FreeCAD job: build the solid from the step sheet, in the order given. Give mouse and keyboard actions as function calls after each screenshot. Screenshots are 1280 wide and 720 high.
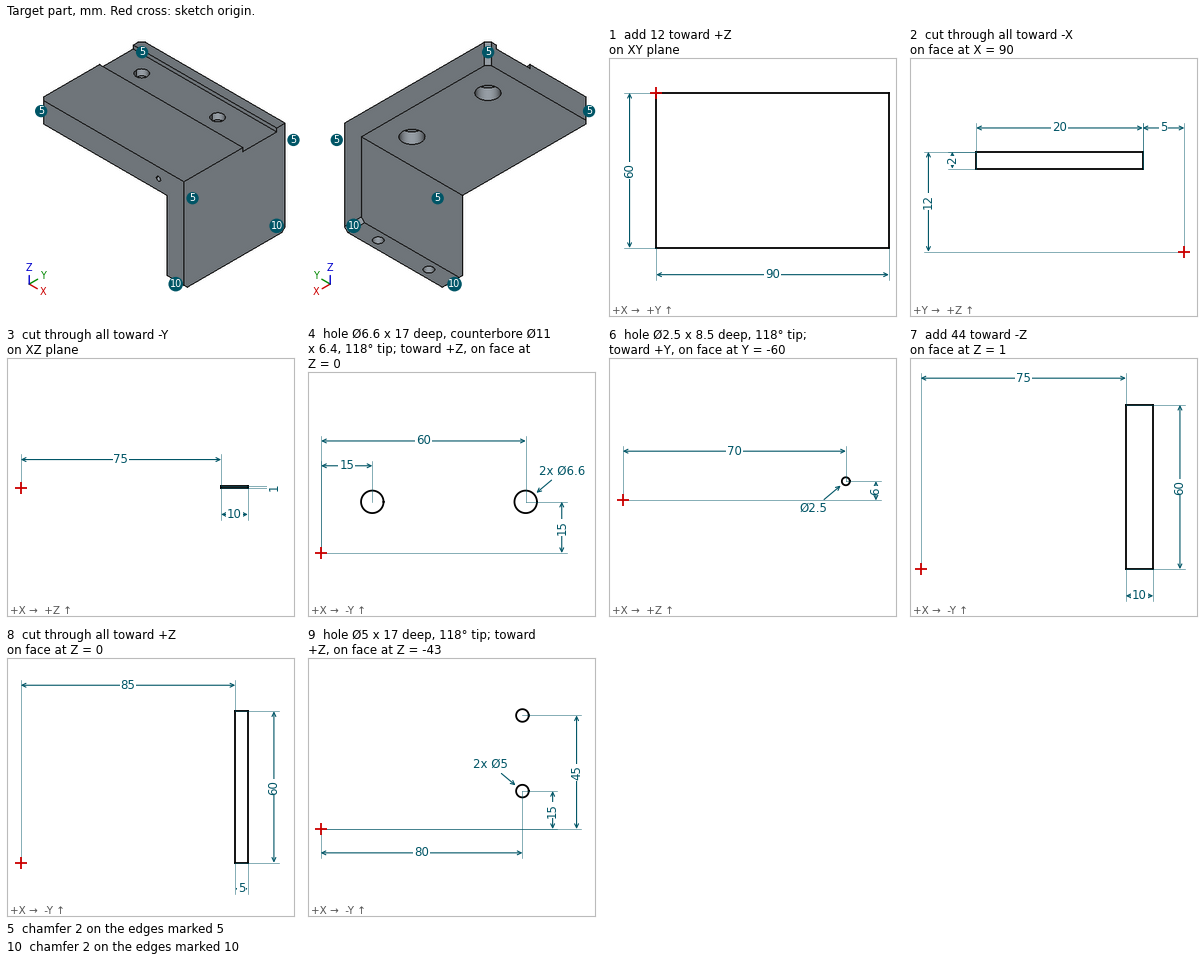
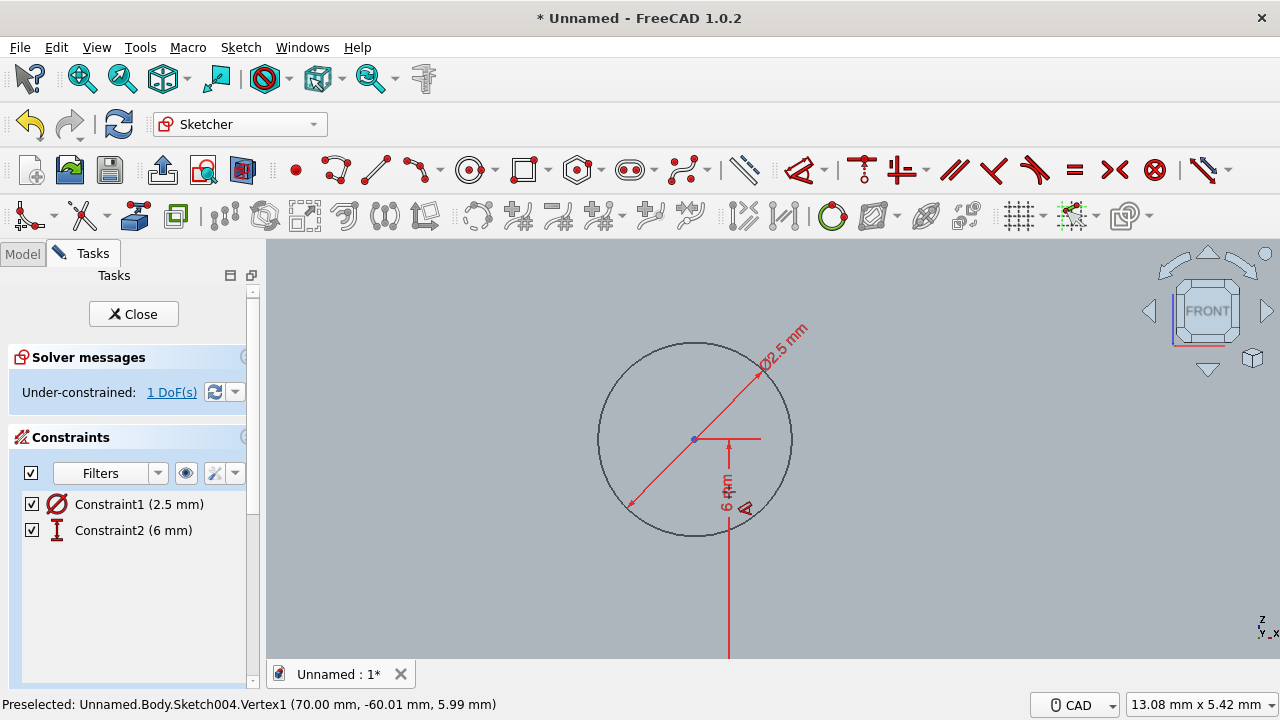
click(695, 439)
click(494, 405)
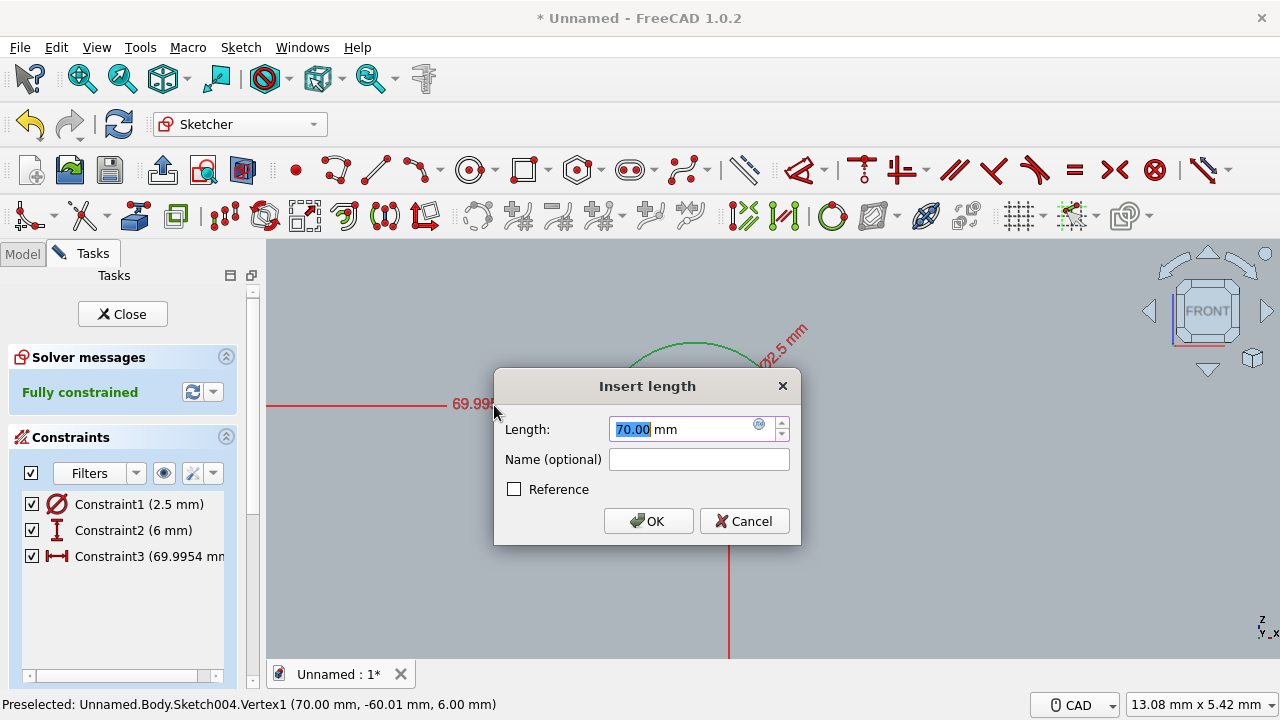
text(70)
key(Return)
key(Escape)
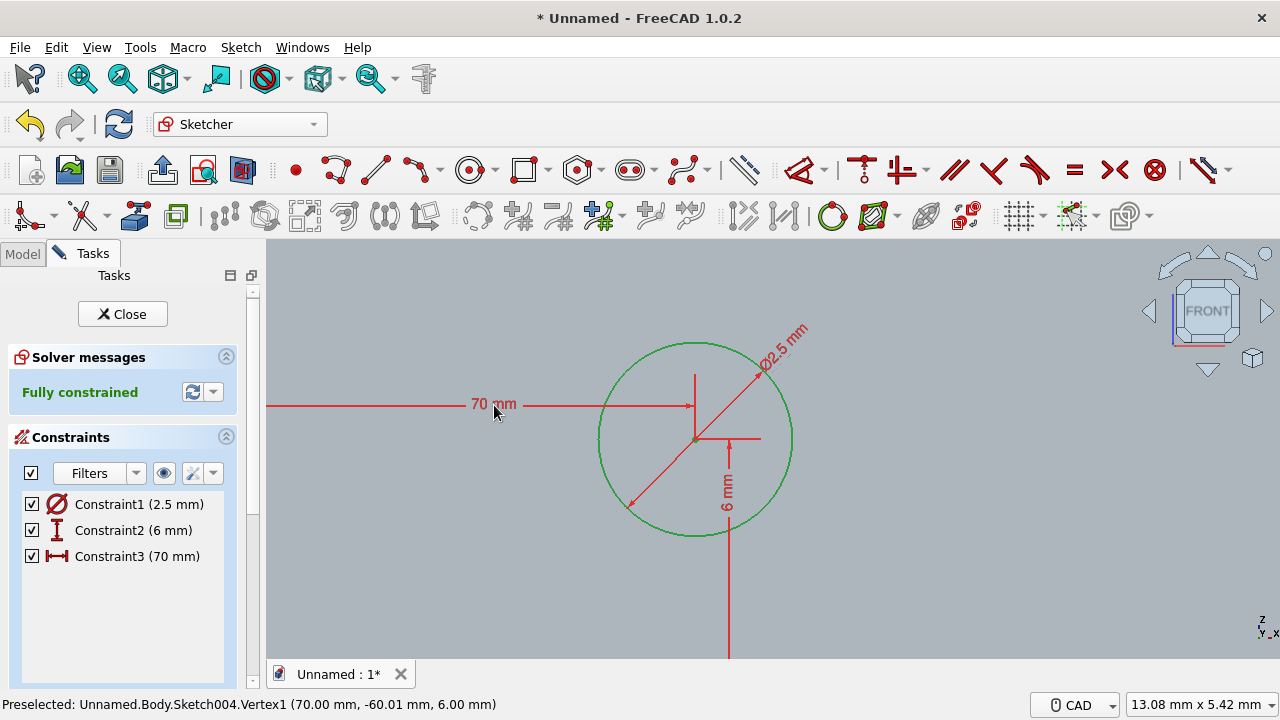
click(123, 314)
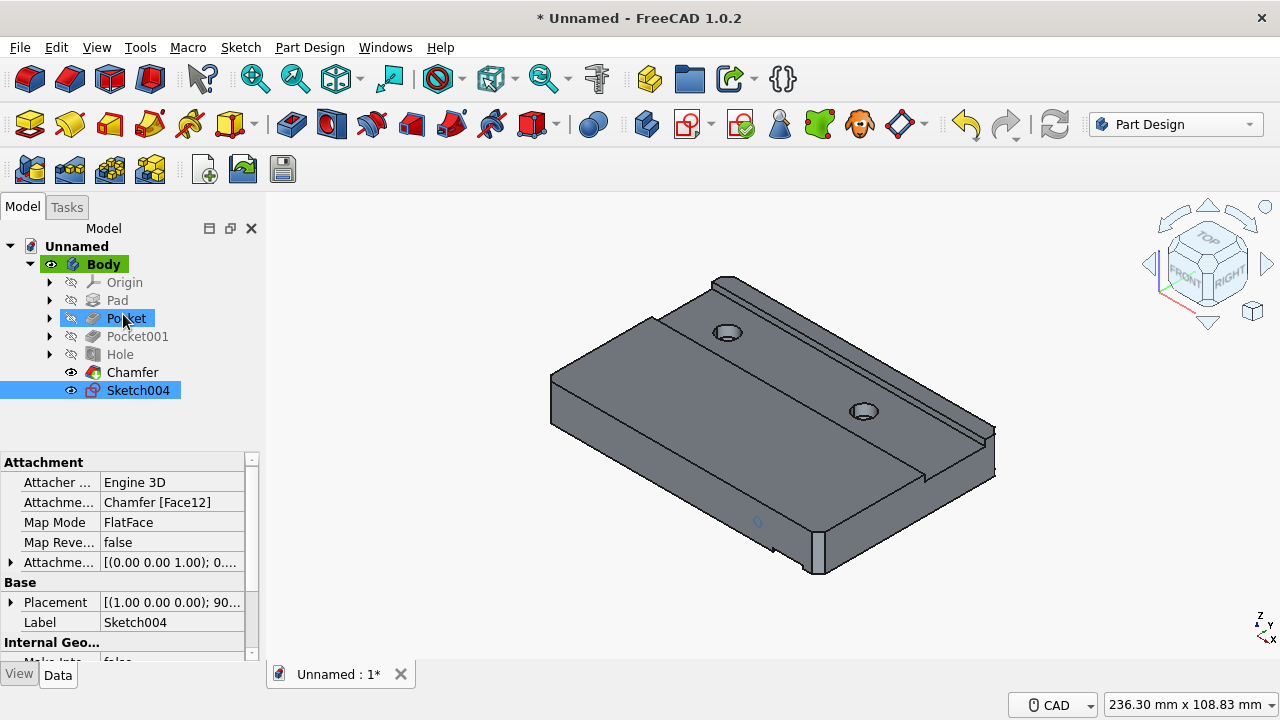
click(332, 124)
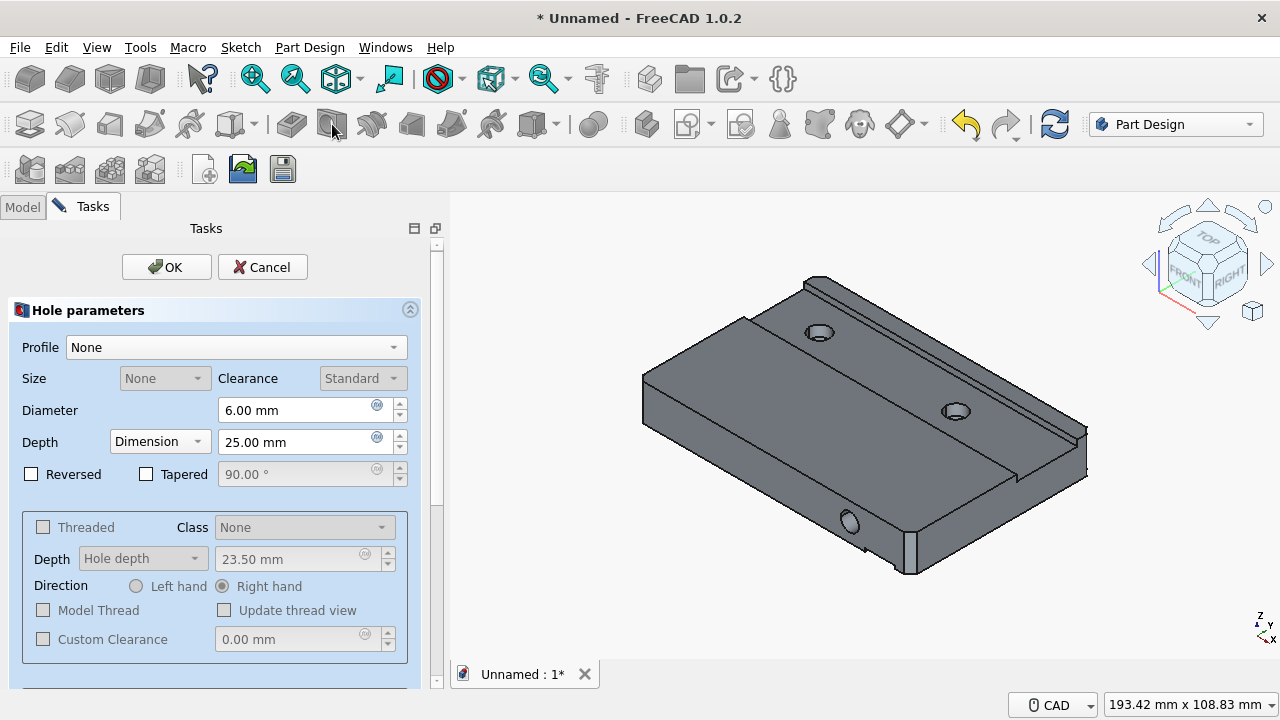
triple_click(305, 410)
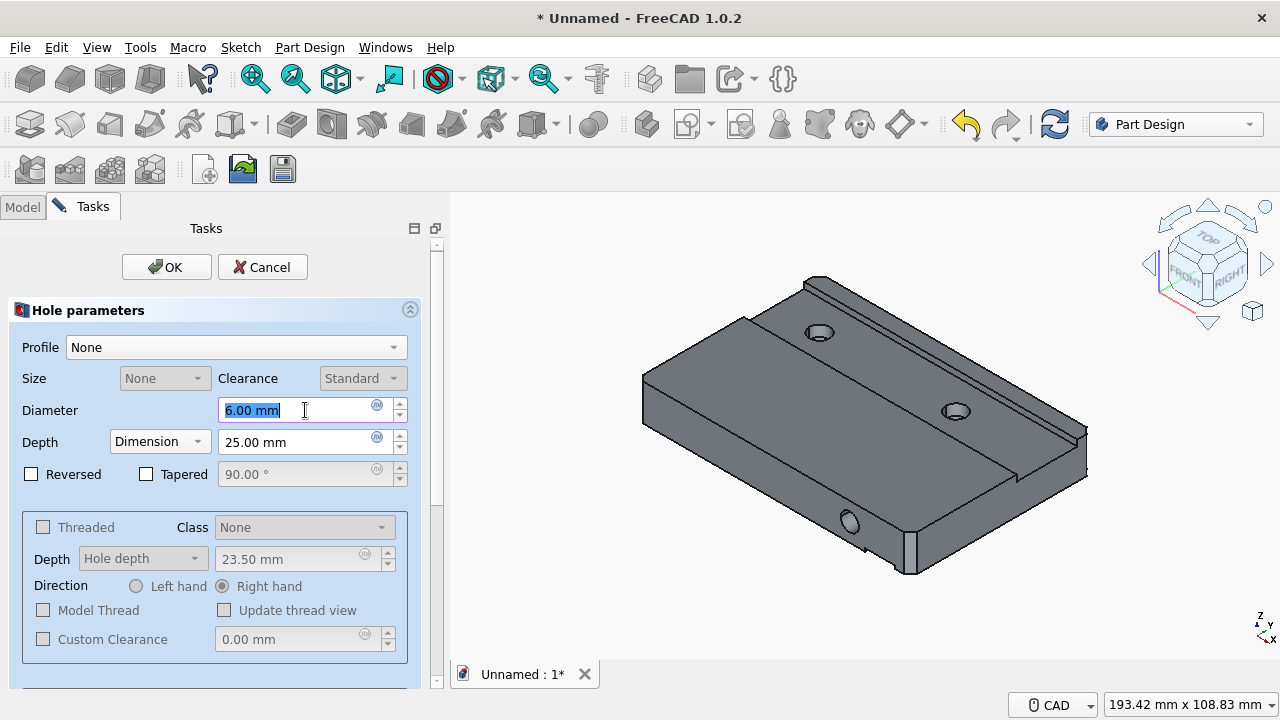
text(2.5)
key(Tab)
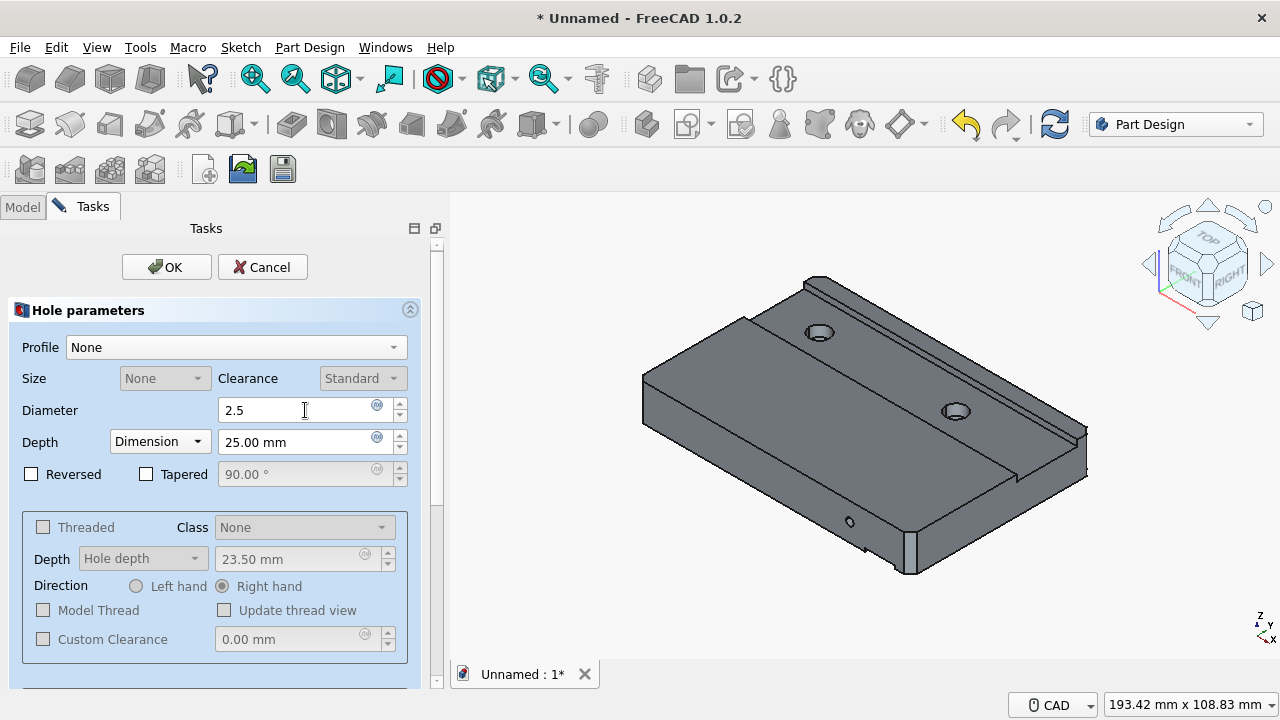
triple_click(305, 442)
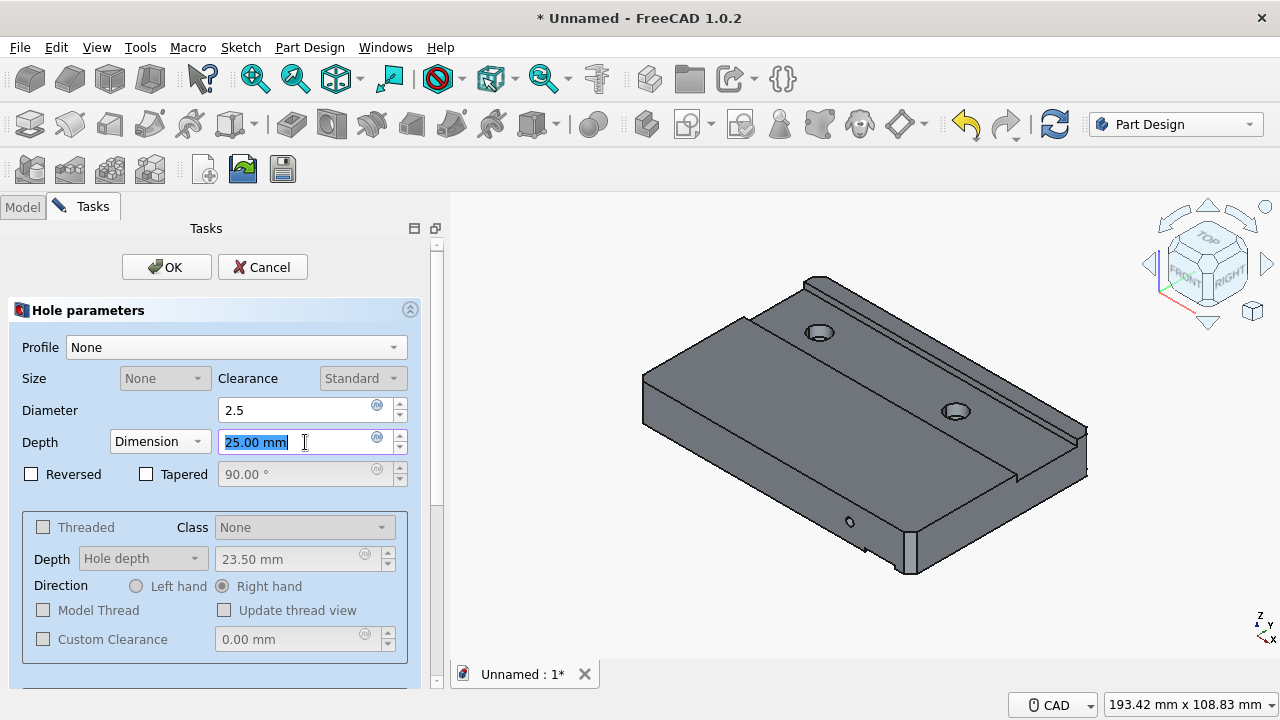
text(8.5)
key(Tab)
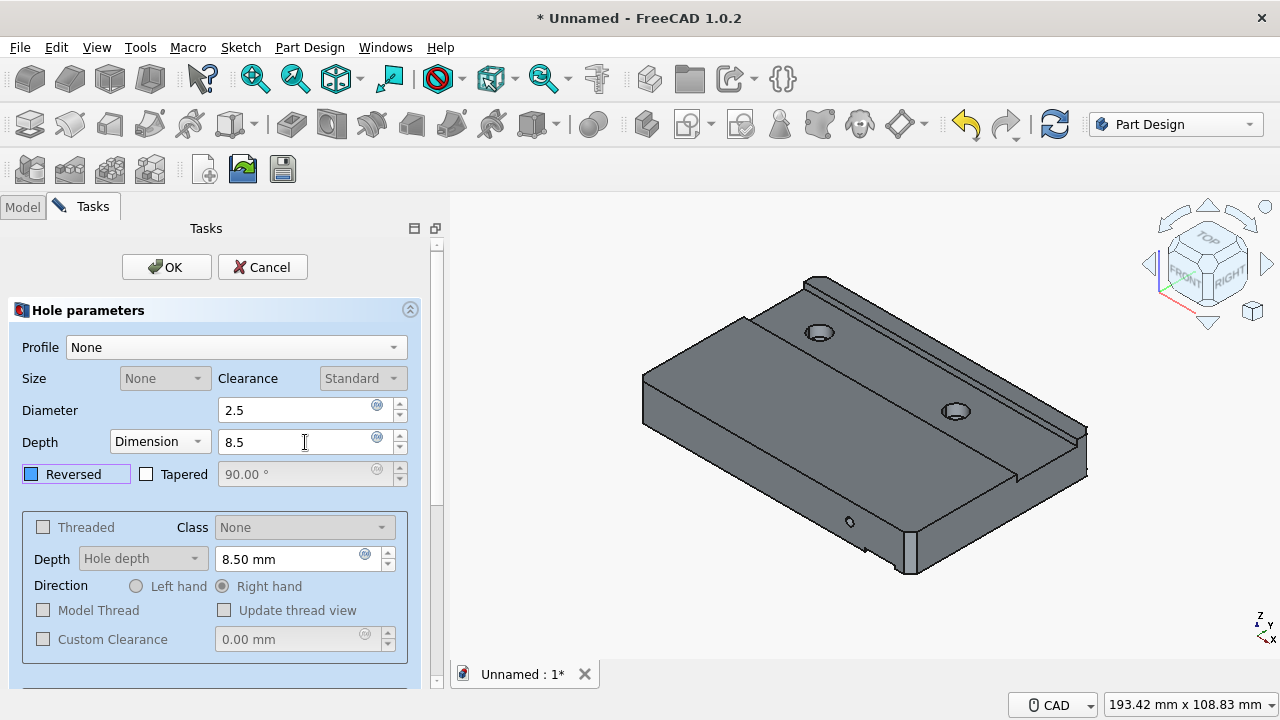
click(167, 267)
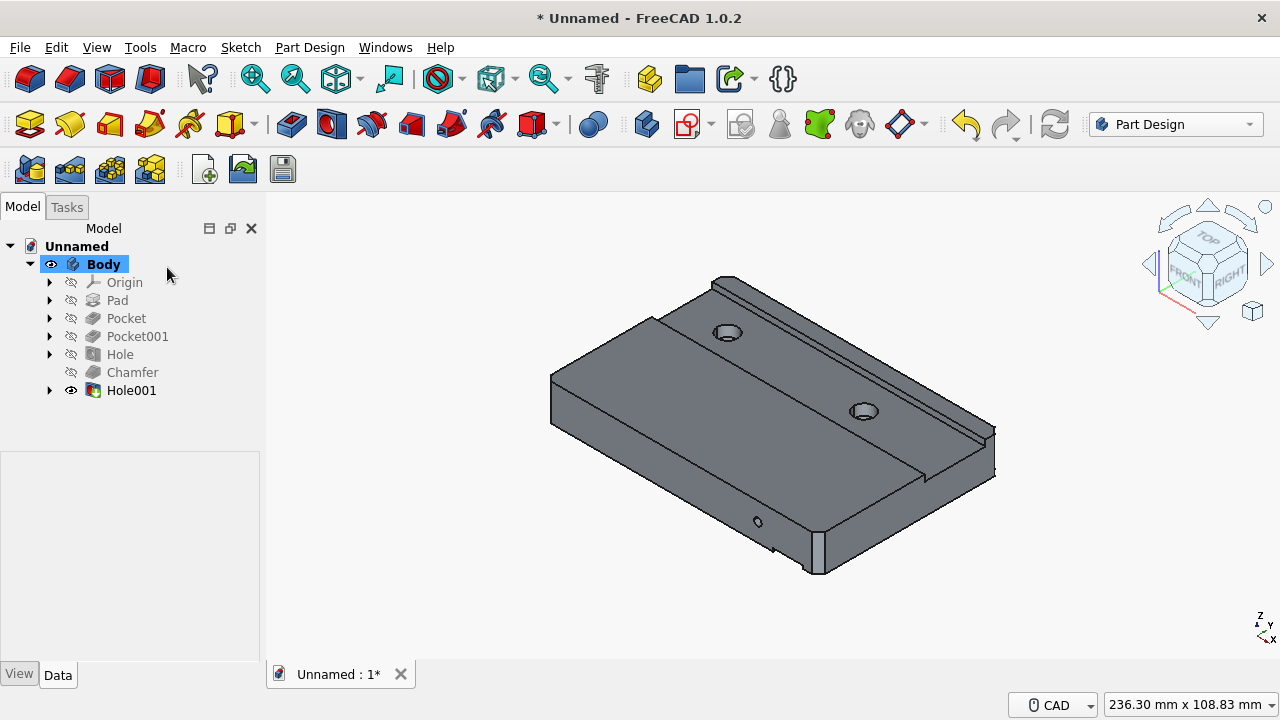
key(5)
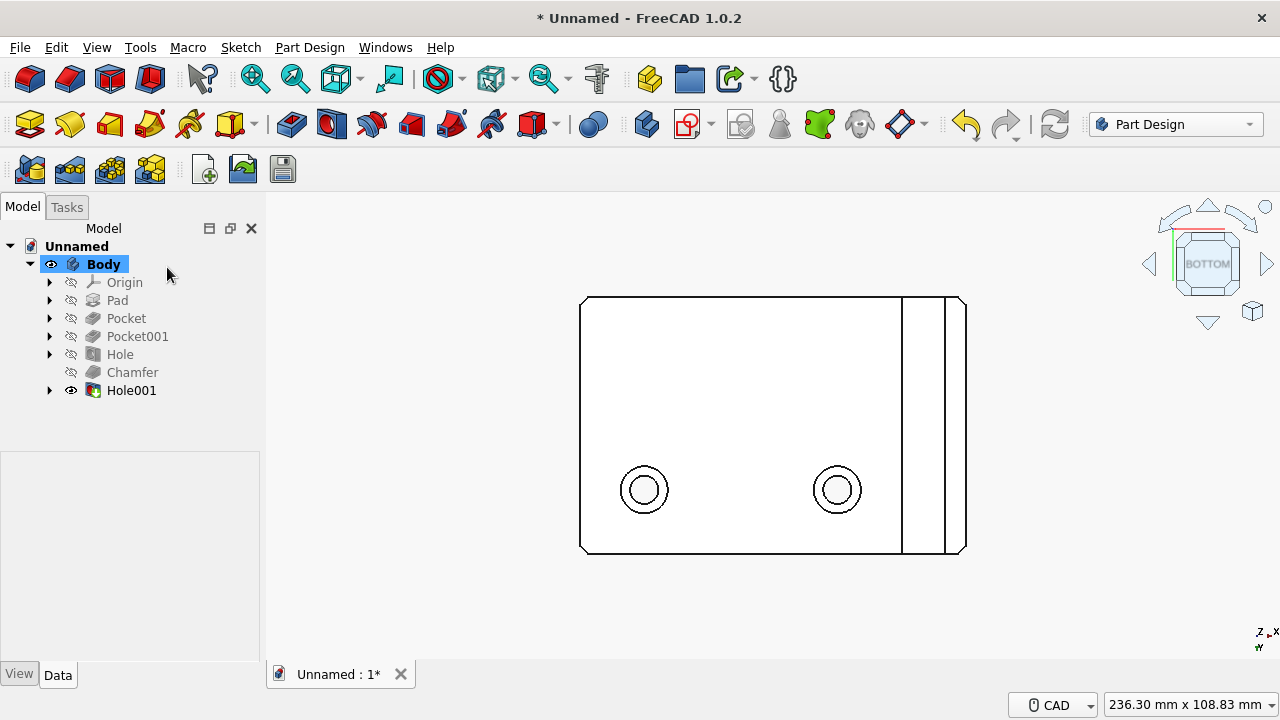
click(923, 498)